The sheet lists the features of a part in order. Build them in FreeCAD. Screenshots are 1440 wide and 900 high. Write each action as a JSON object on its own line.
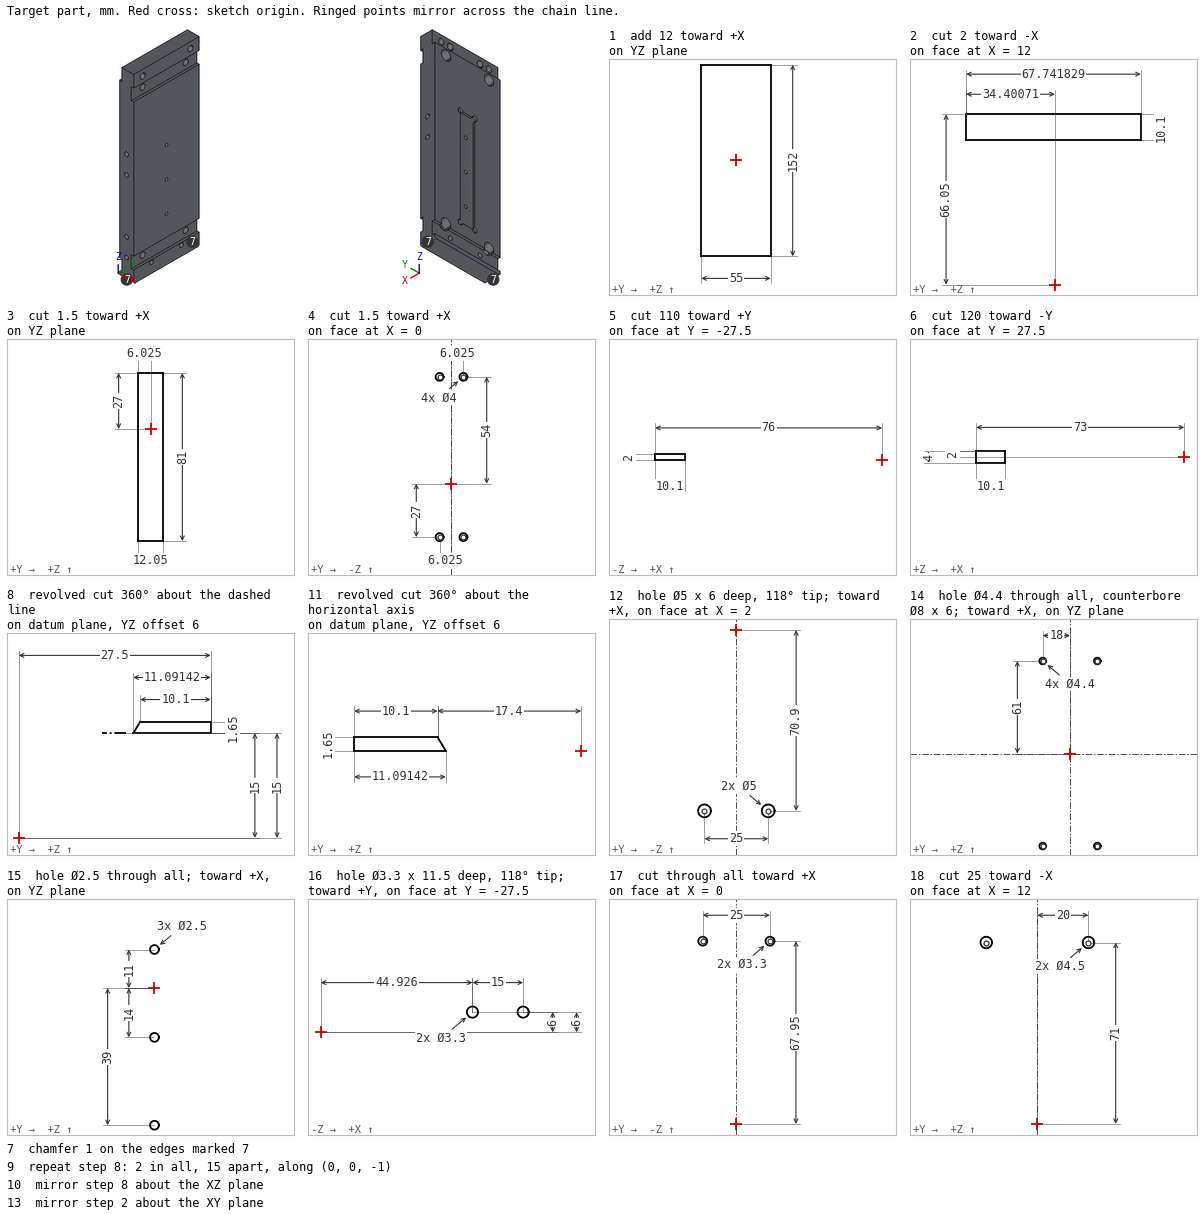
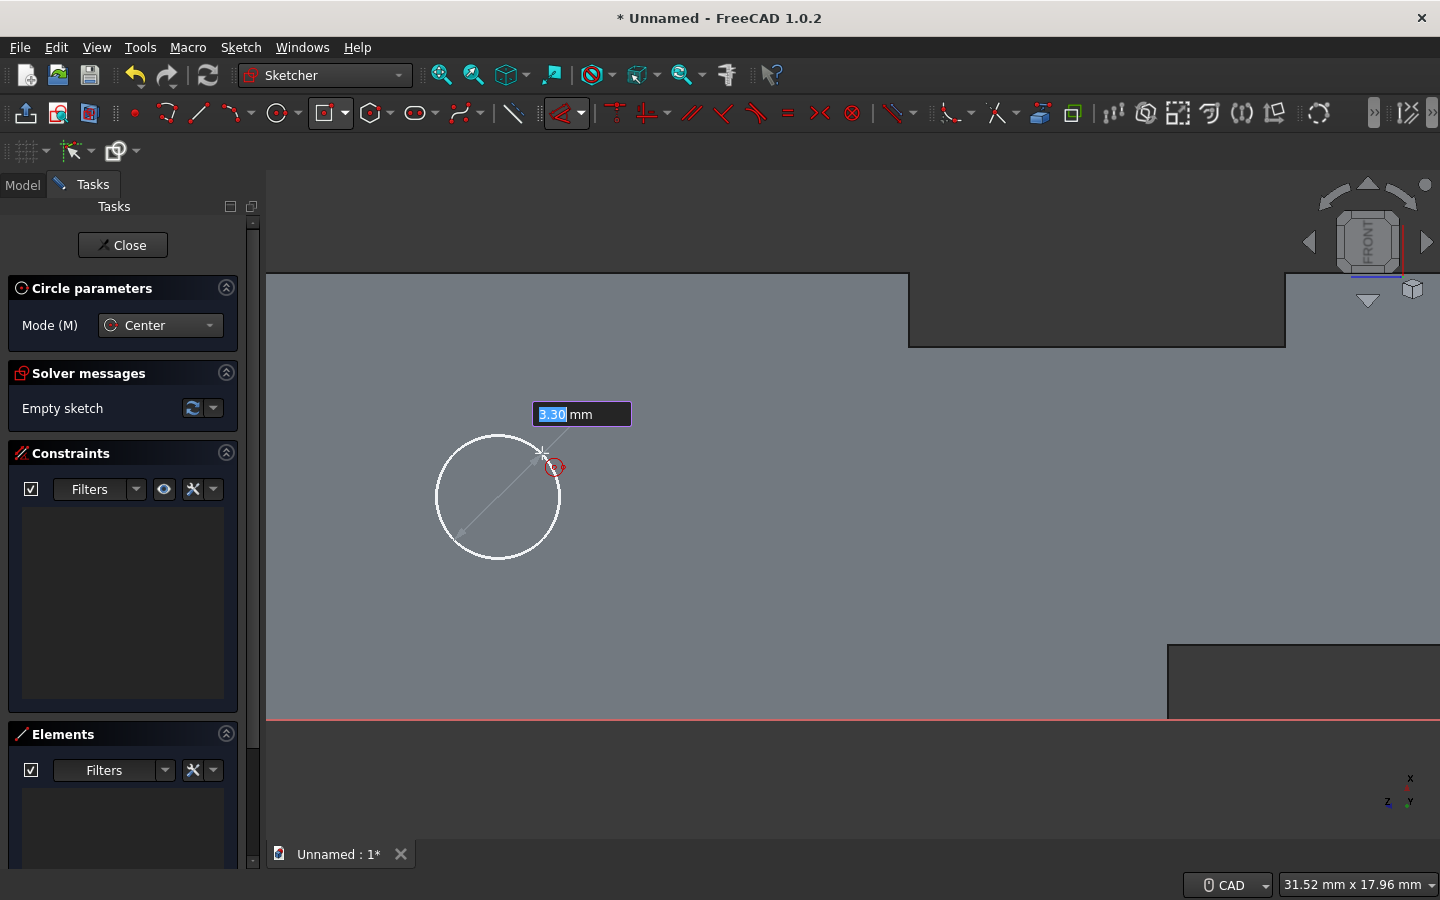
{"action": "type", "text": "3.3"}
{"action": "key", "text": "Return"}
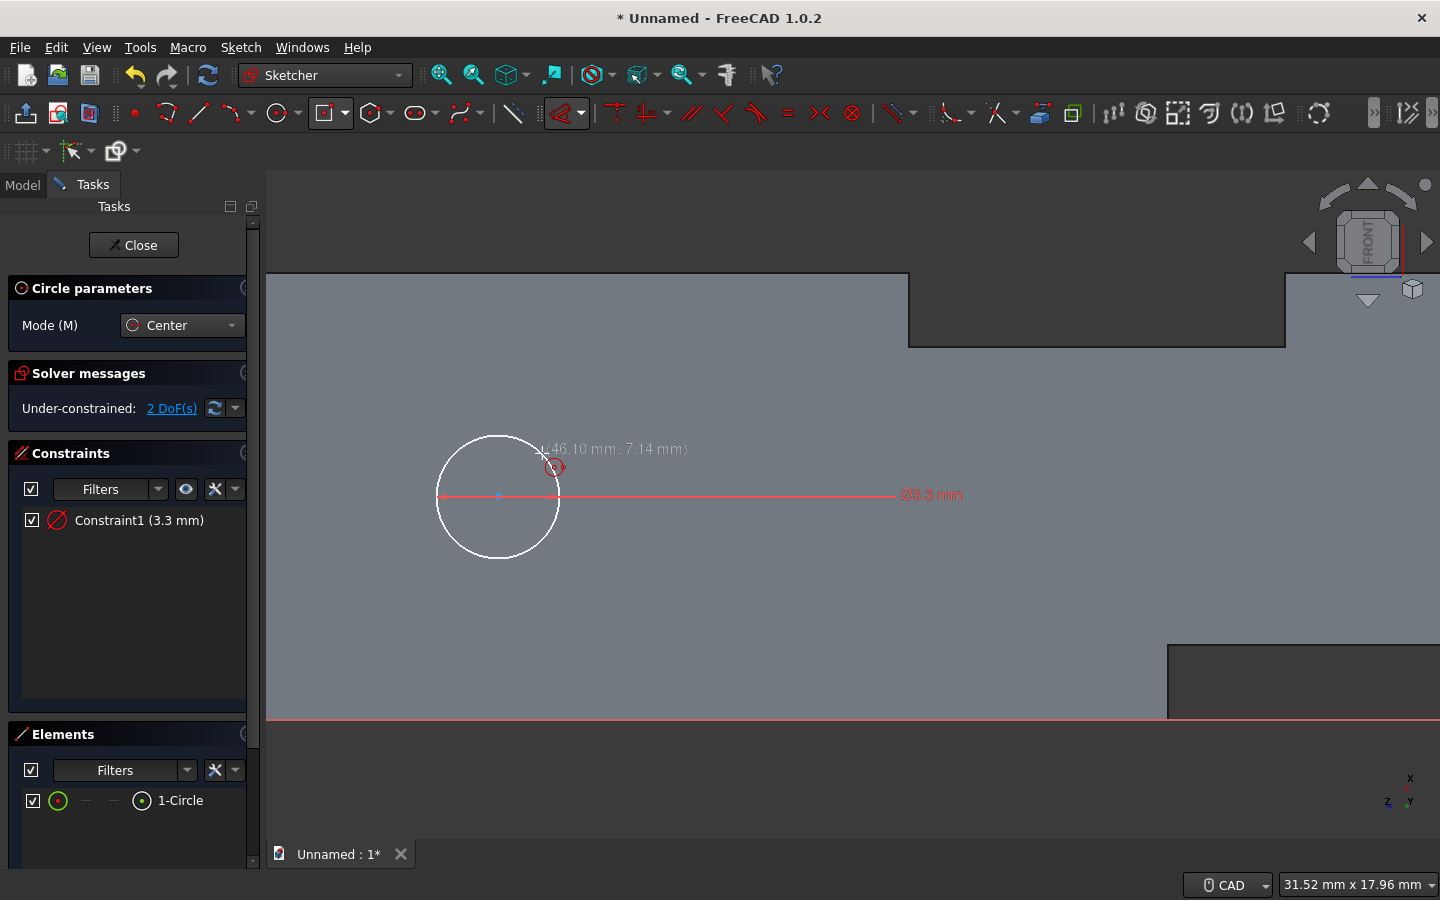
{"action": "left_click", "coordinate": [1057, 496]}
{"action": "mouse_move", "coordinate": [1101, 453]}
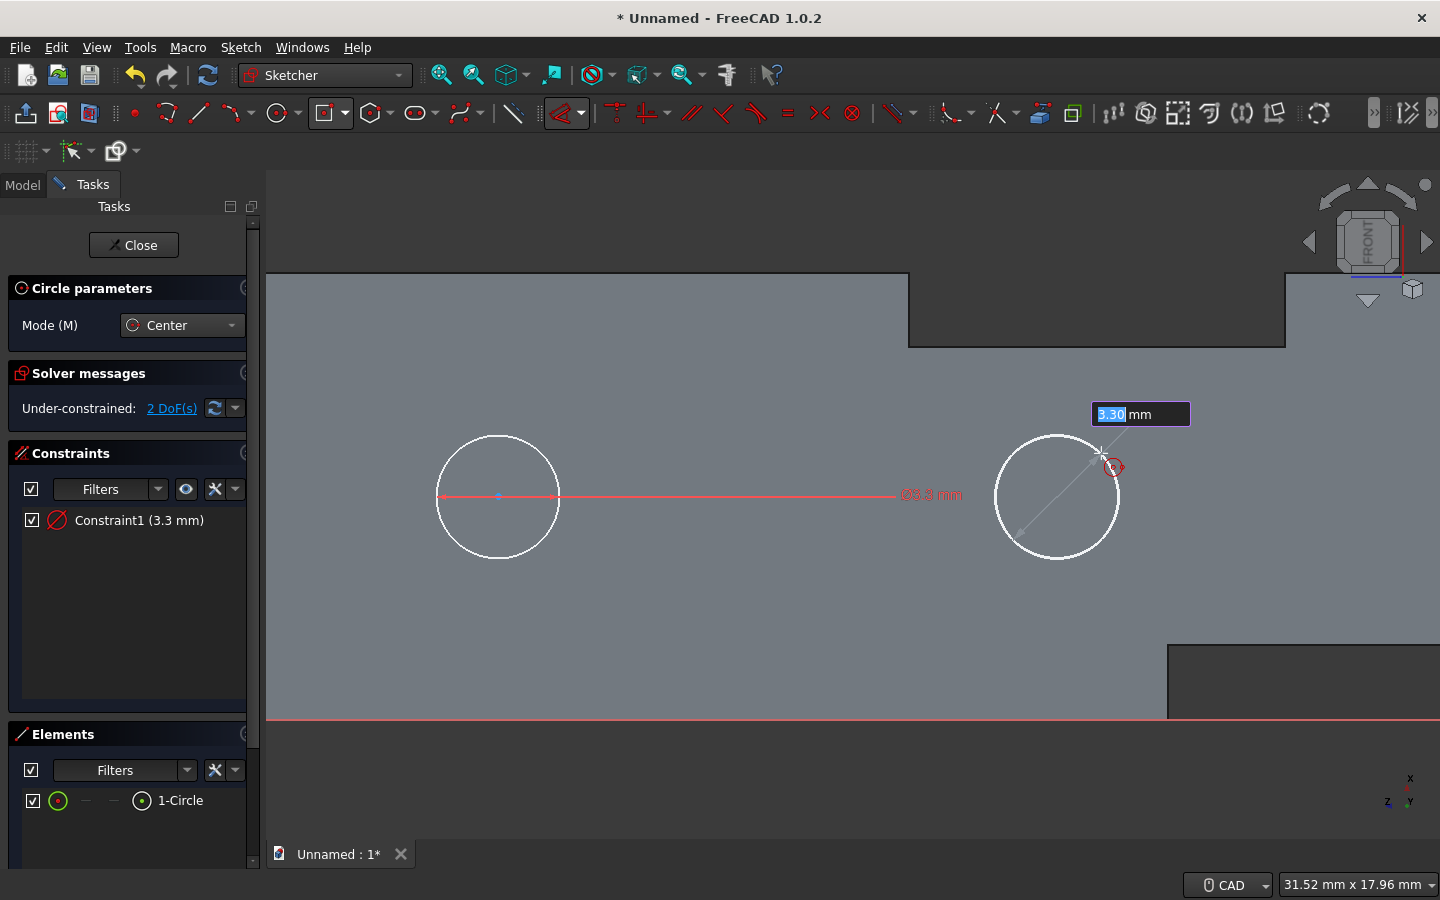
{"action": "type", "text": "3.3"}
{"action": "key", "text": "Return"}
{"action": "key", "text": "Escape"}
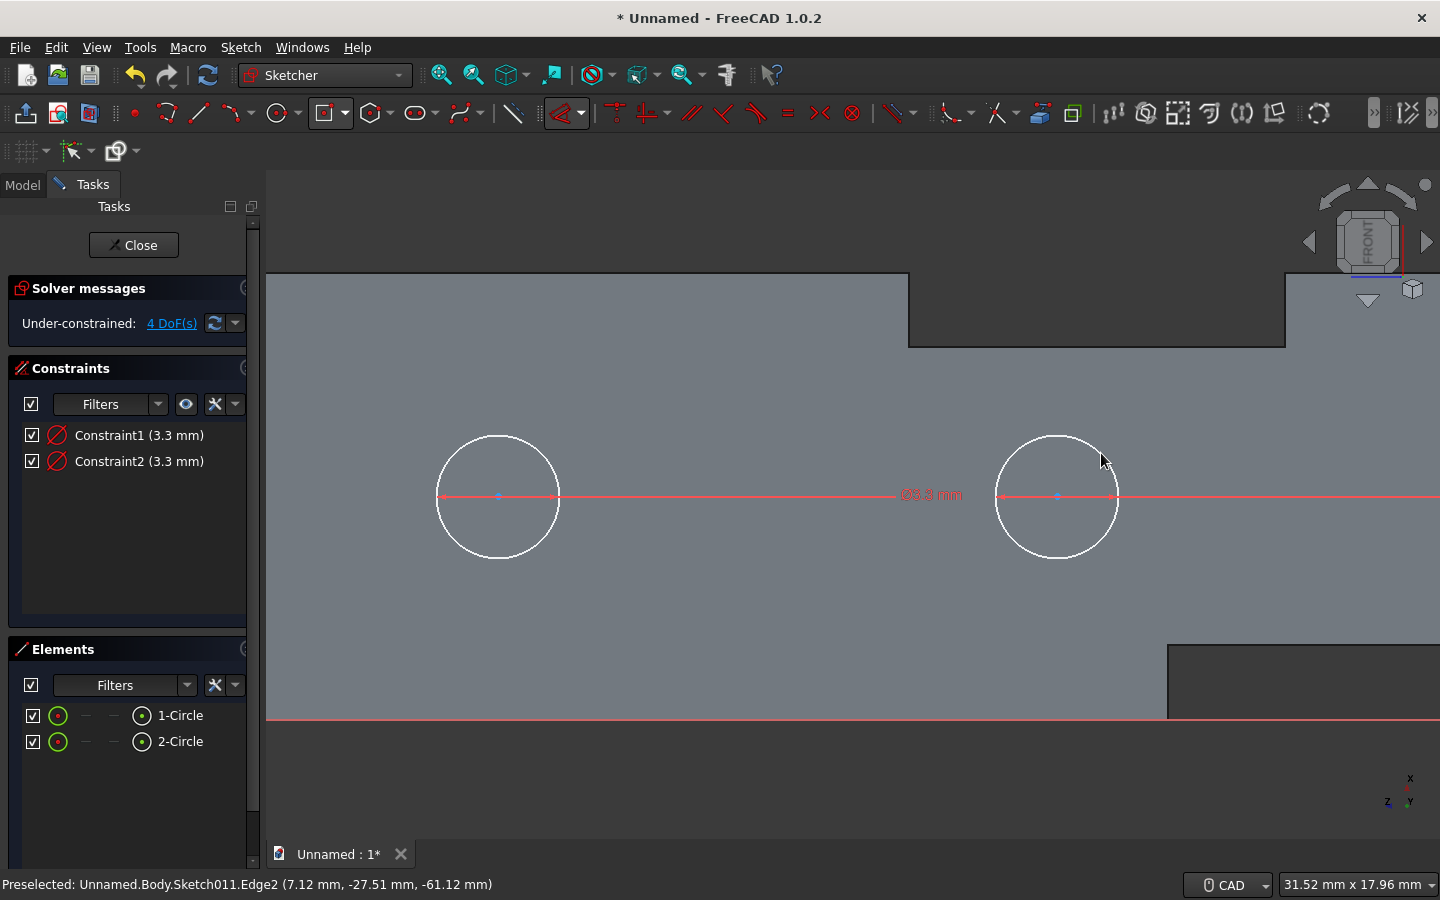
{"action": "left_click", "coordinate": [498, 497]}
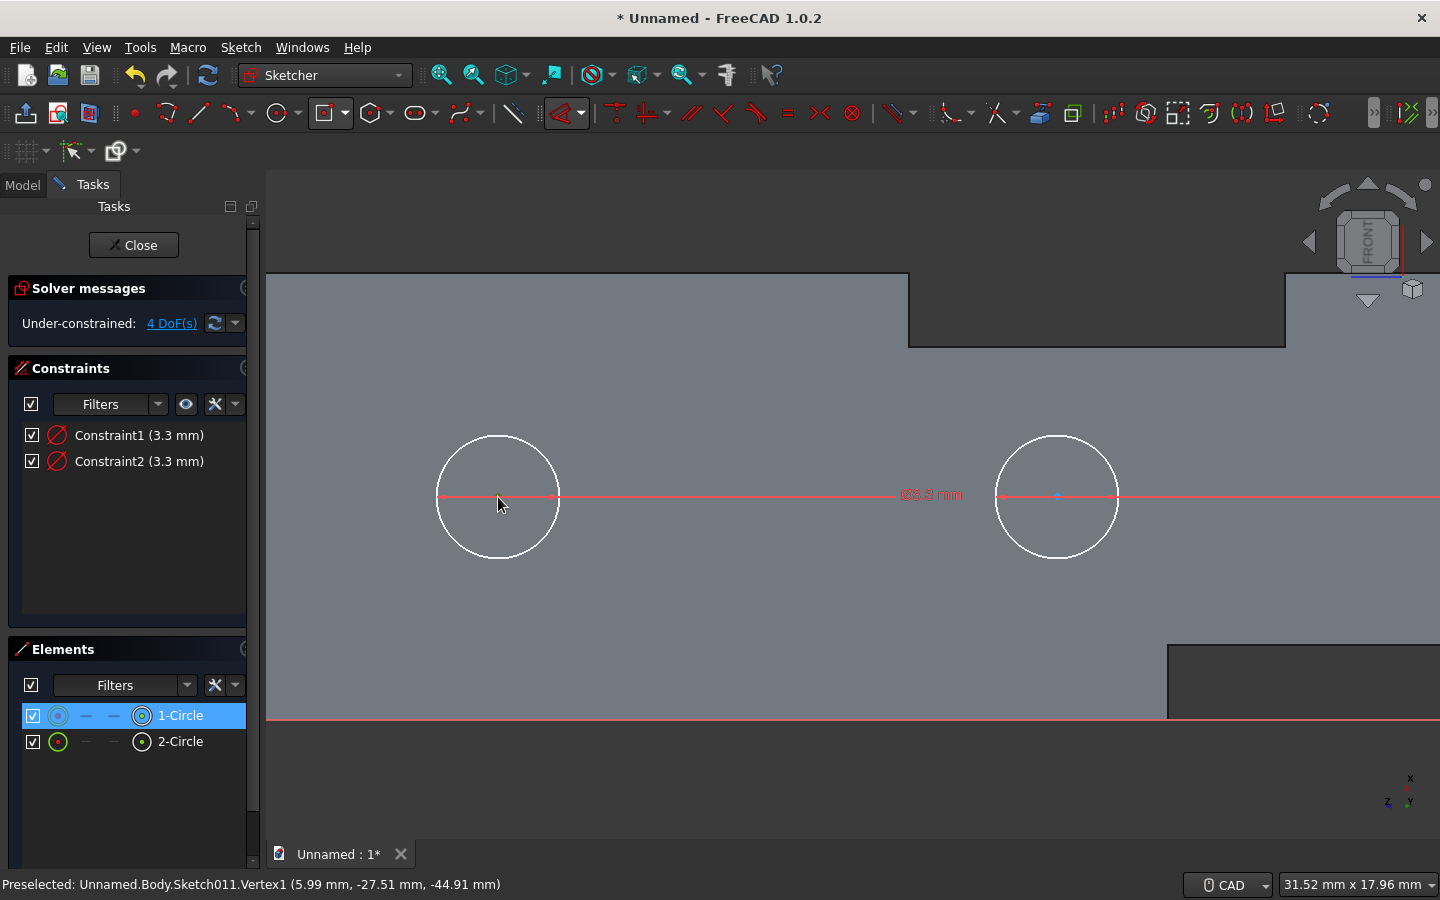
{"action": "left_click", "coordinate": [584, 114]}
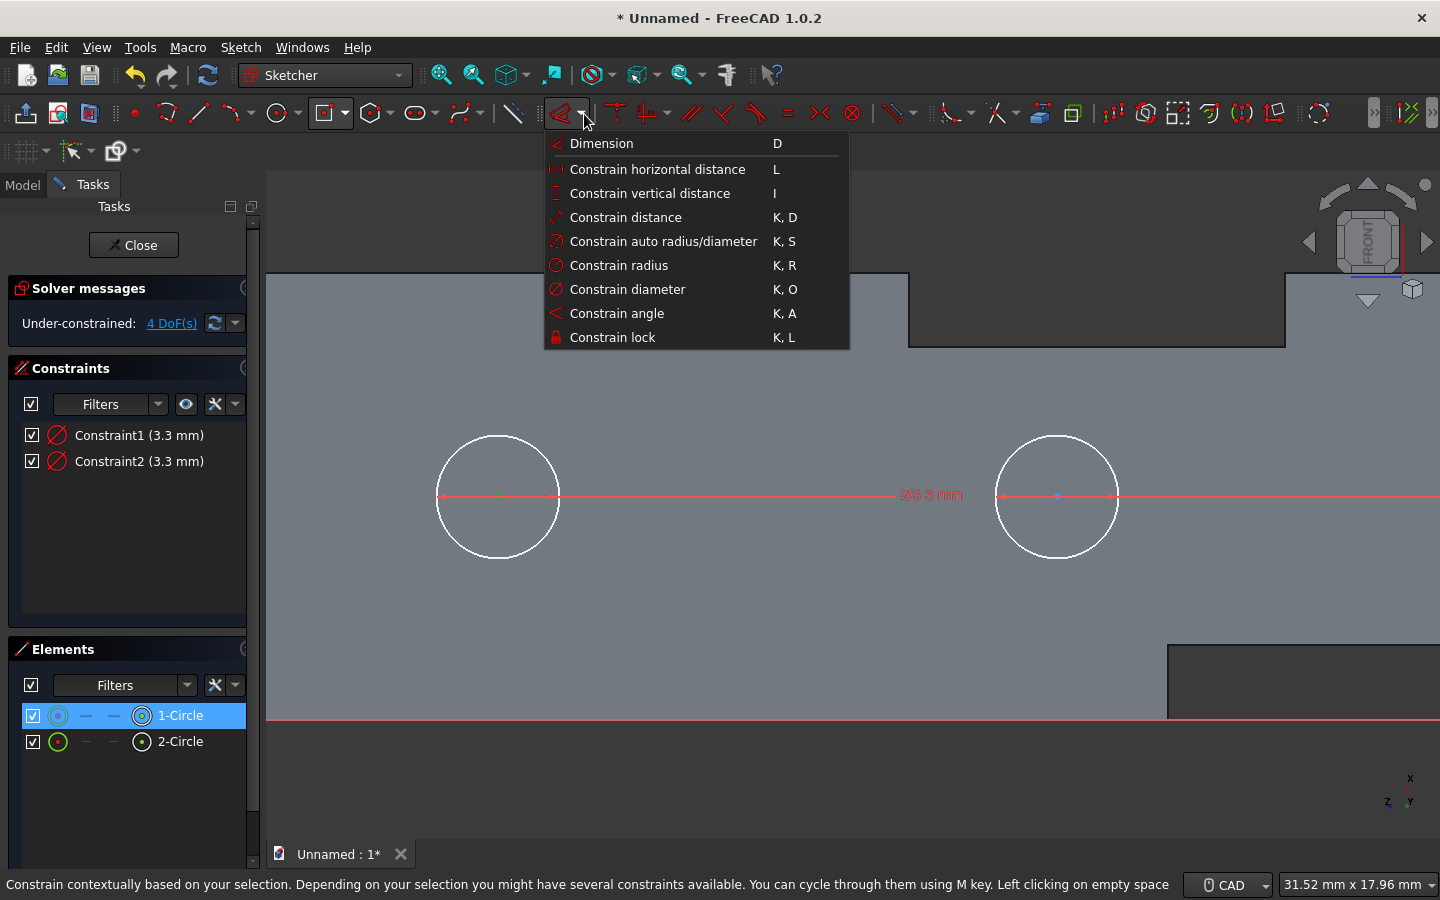
{"action": "left_click", "coordinate": [697, 193]}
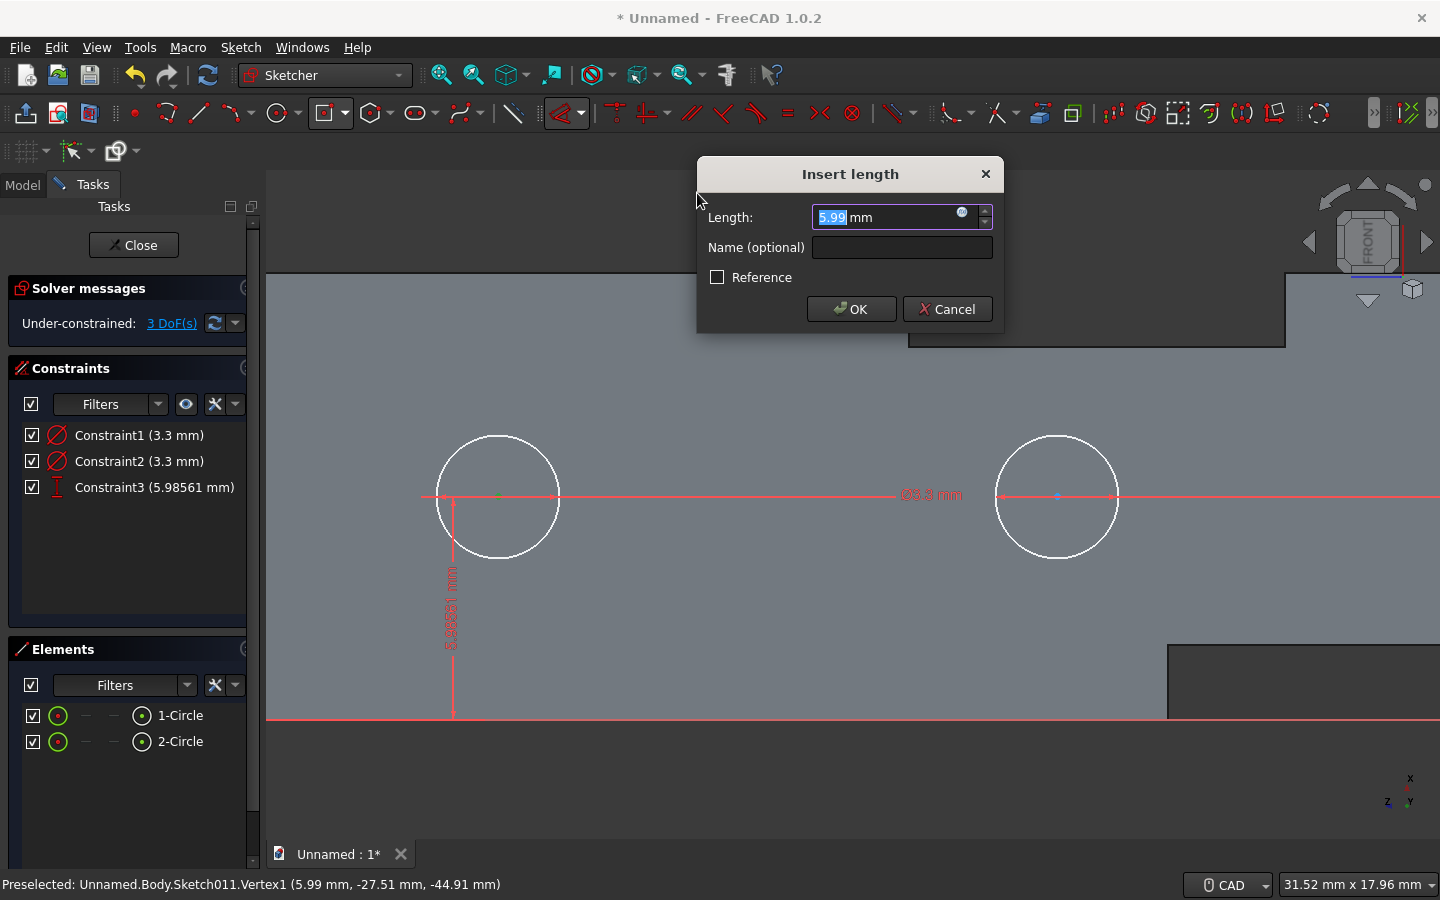
{"action": "type", "text": "6"}
{"action": "key", "text": "Return"}